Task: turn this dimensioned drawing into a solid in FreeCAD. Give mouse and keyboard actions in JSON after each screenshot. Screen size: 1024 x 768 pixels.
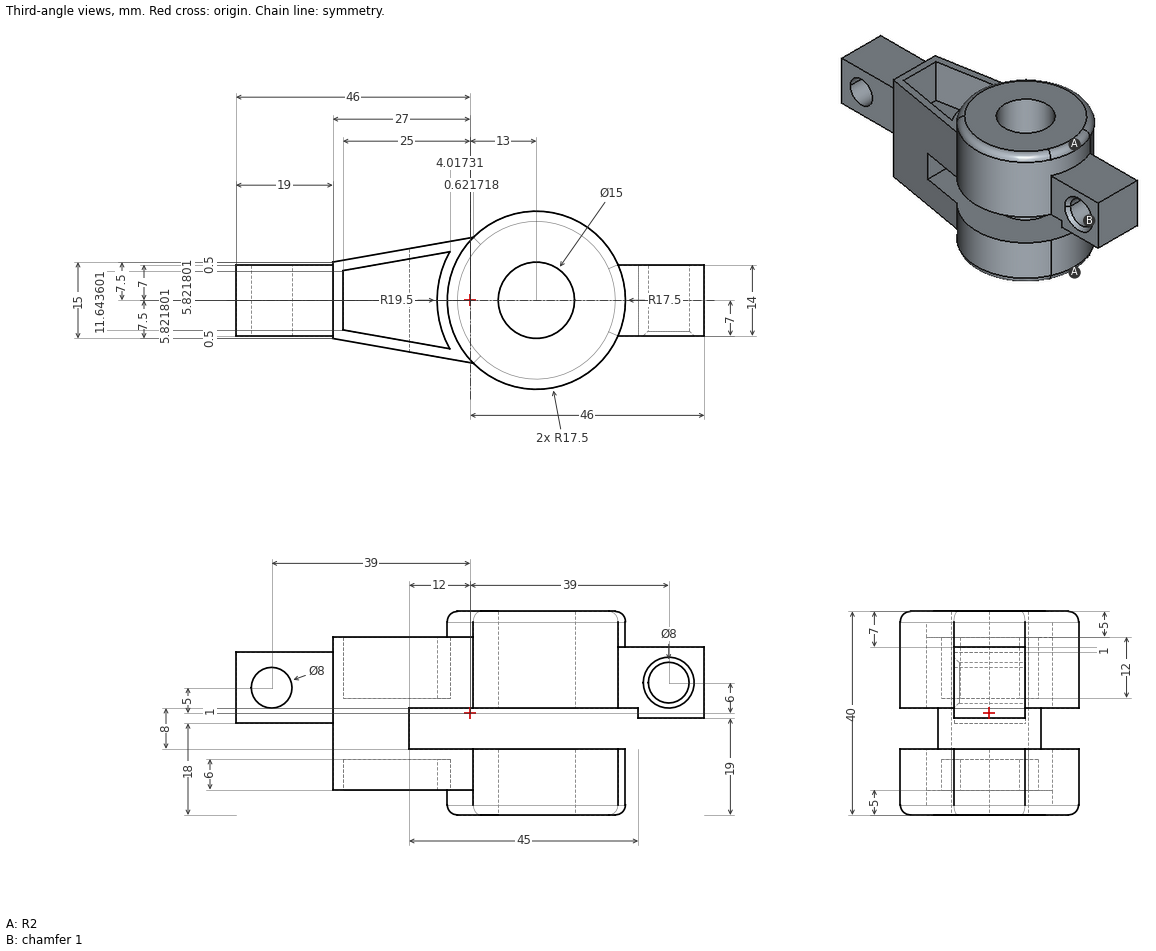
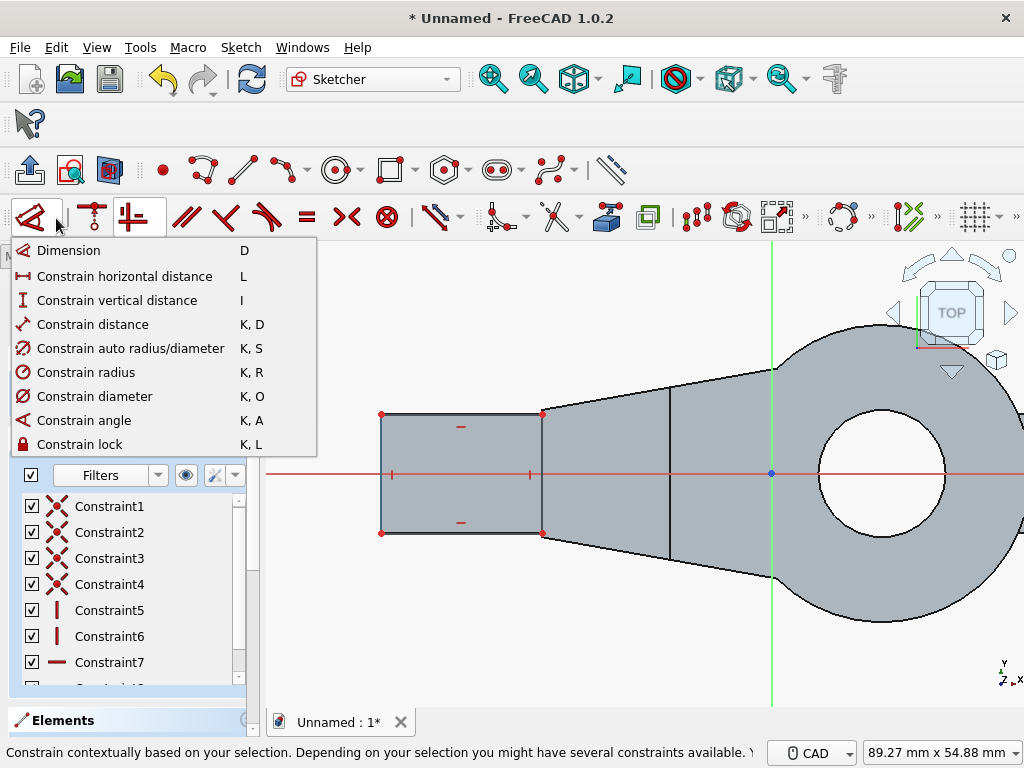
{"action": "left_click", "coordinate": [164, 300]}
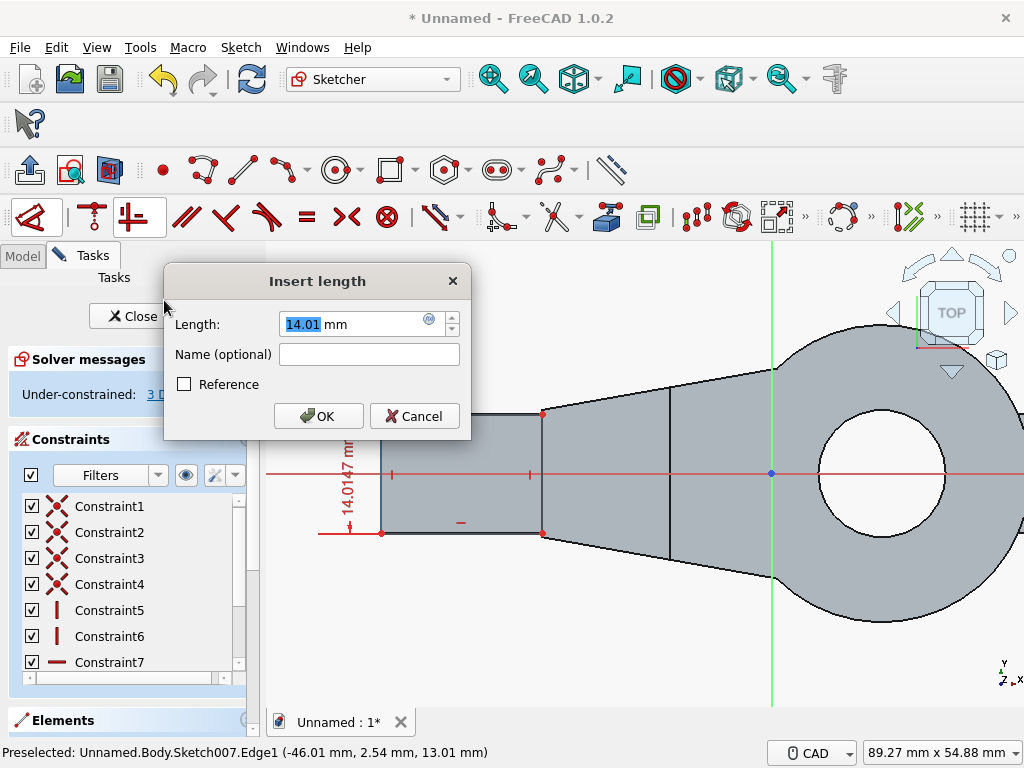
{"action": "type", "text": "14"}
{"action": "key", "text": "Return"}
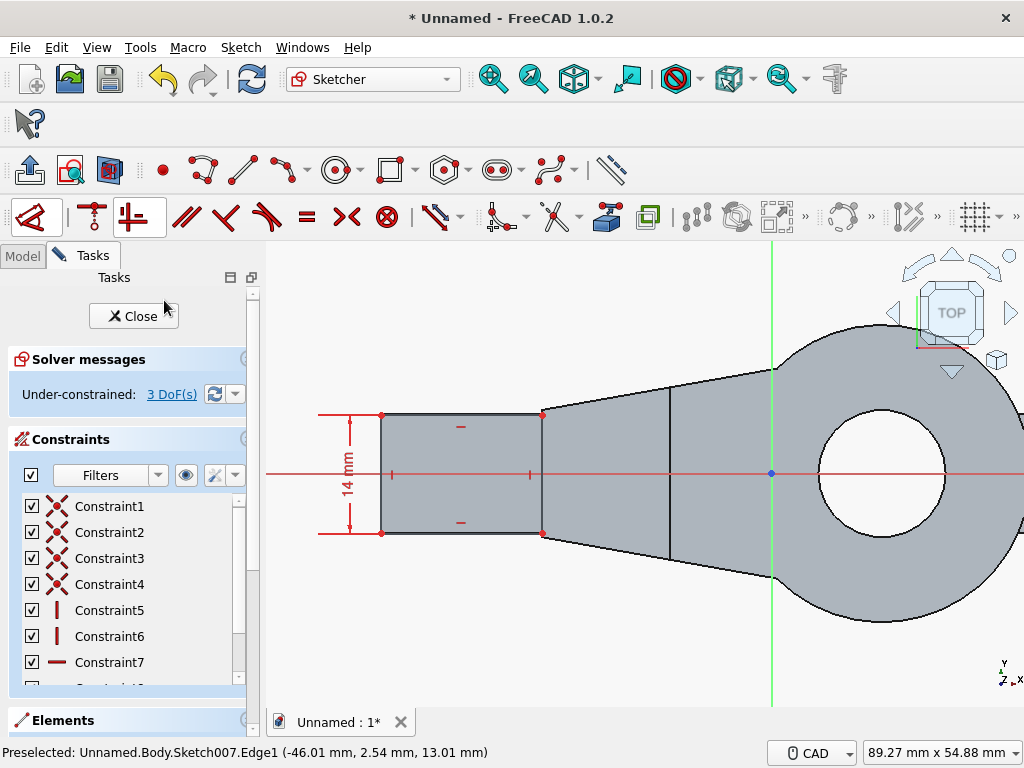
{"action": "left_click", "coordinate": [429, 534]}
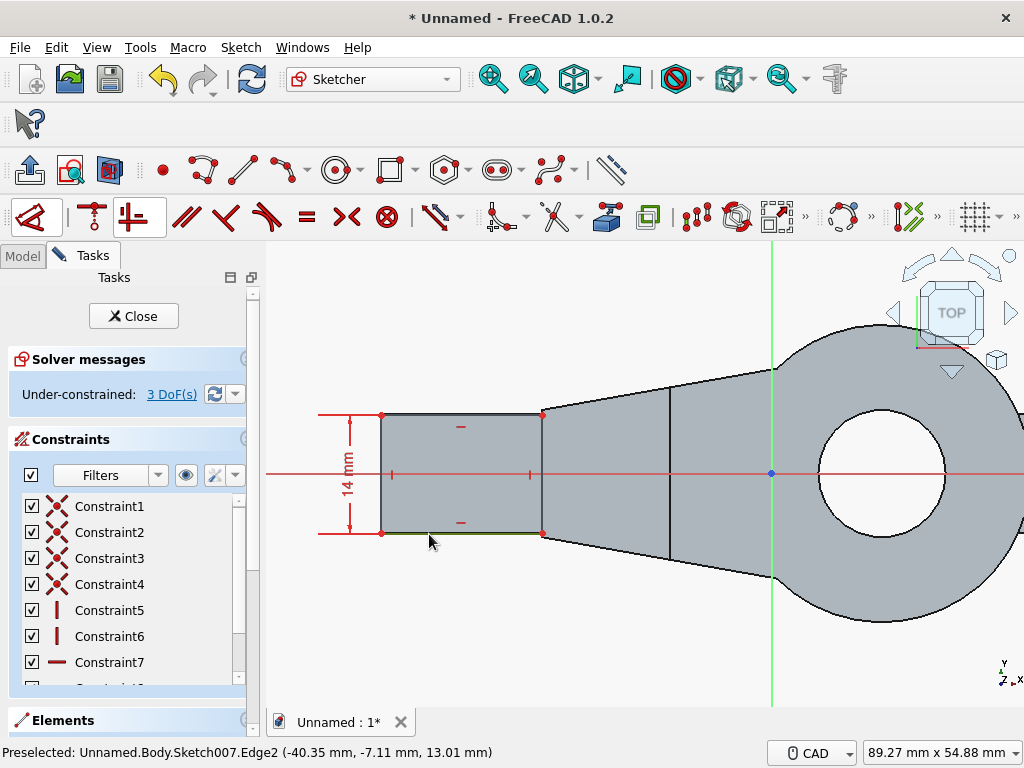
{"action": "key", "text": "l"}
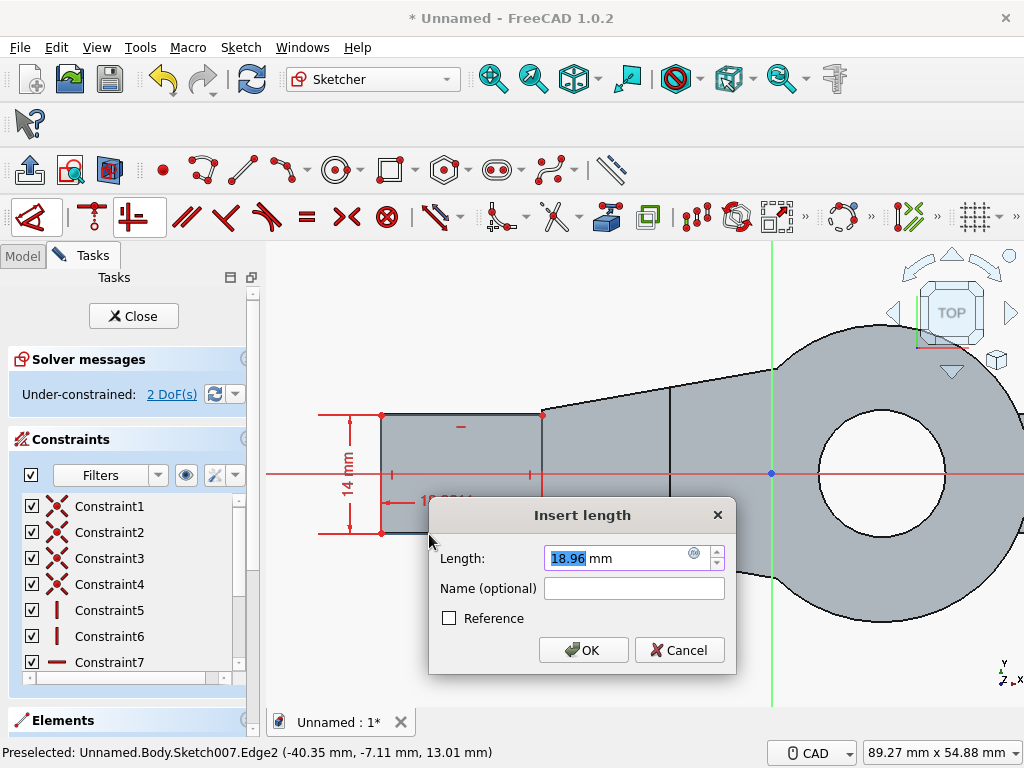
{"action": "type", "text": "19"}
{"action": "key", "text": "Return"}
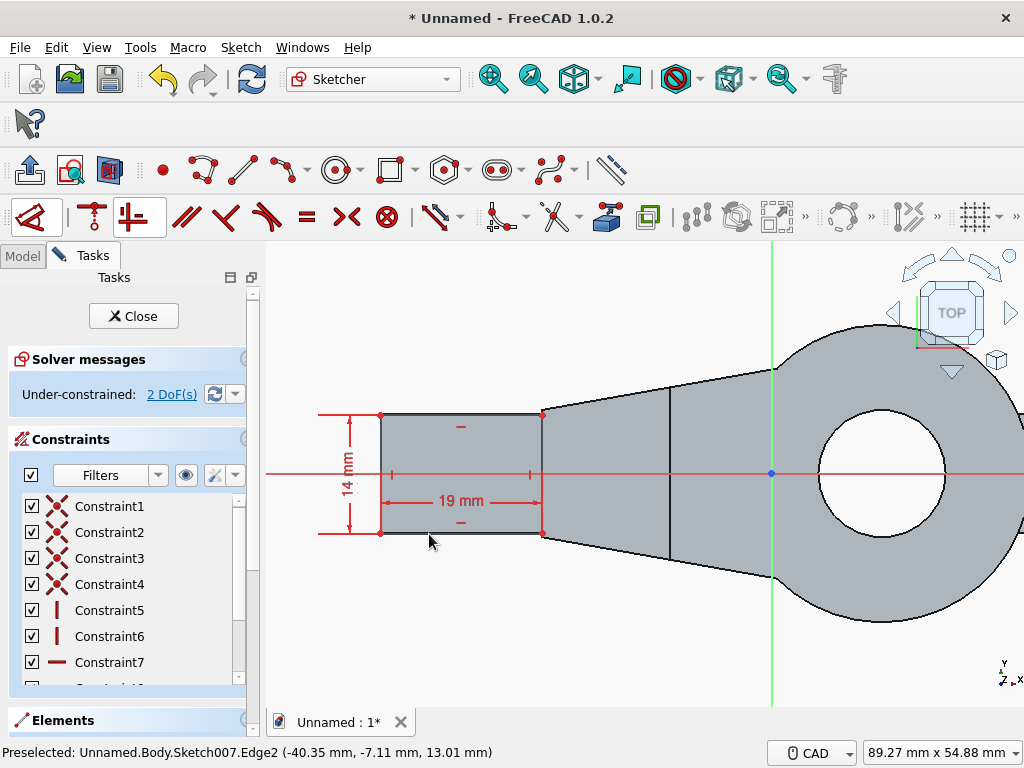
{"action": "left_click", "coordinate": [381, 415]}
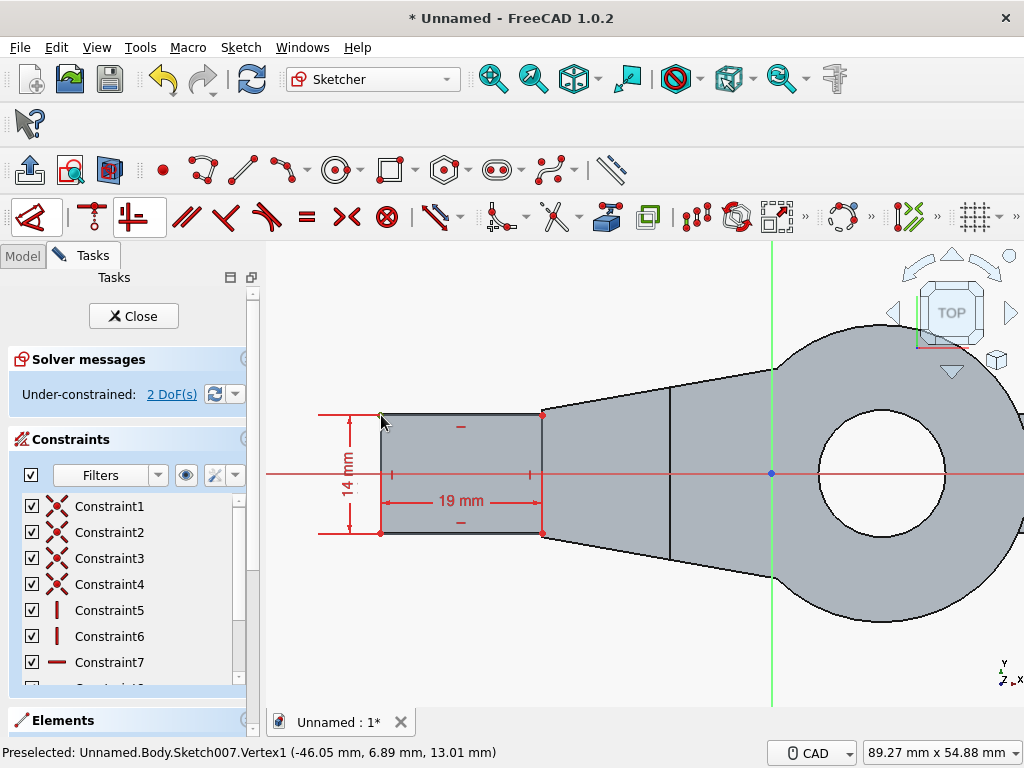
{"action": "left_click", "coordinate": [56, 218]}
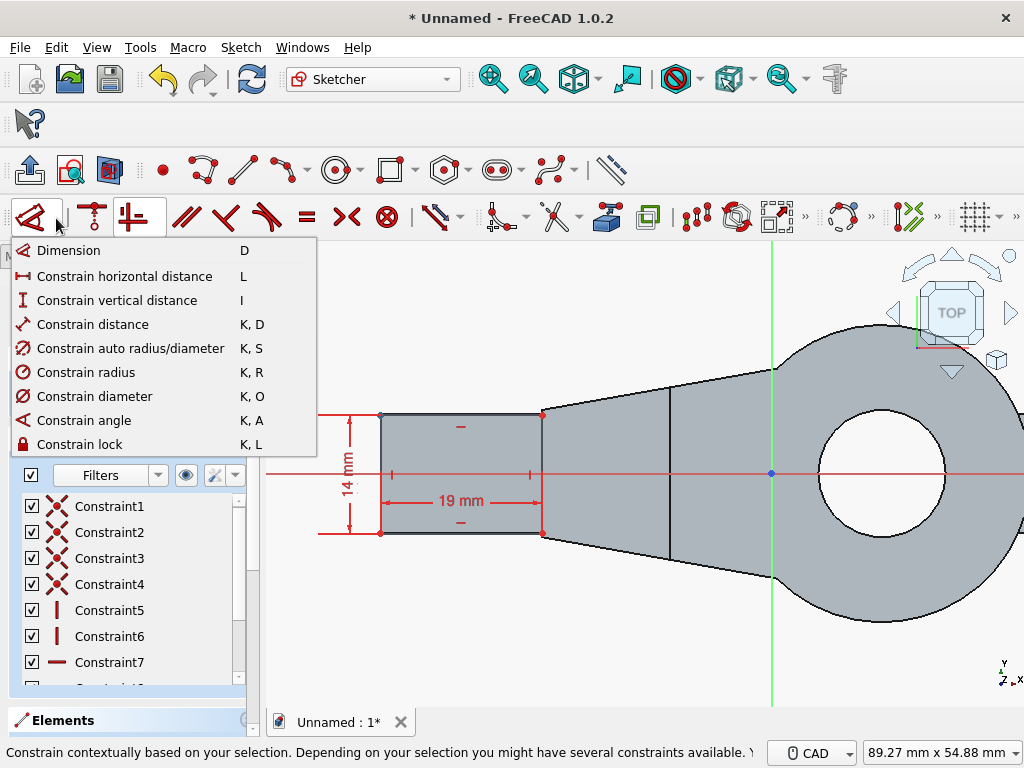
{"action": "left_click", "coordinate": [164, 300]}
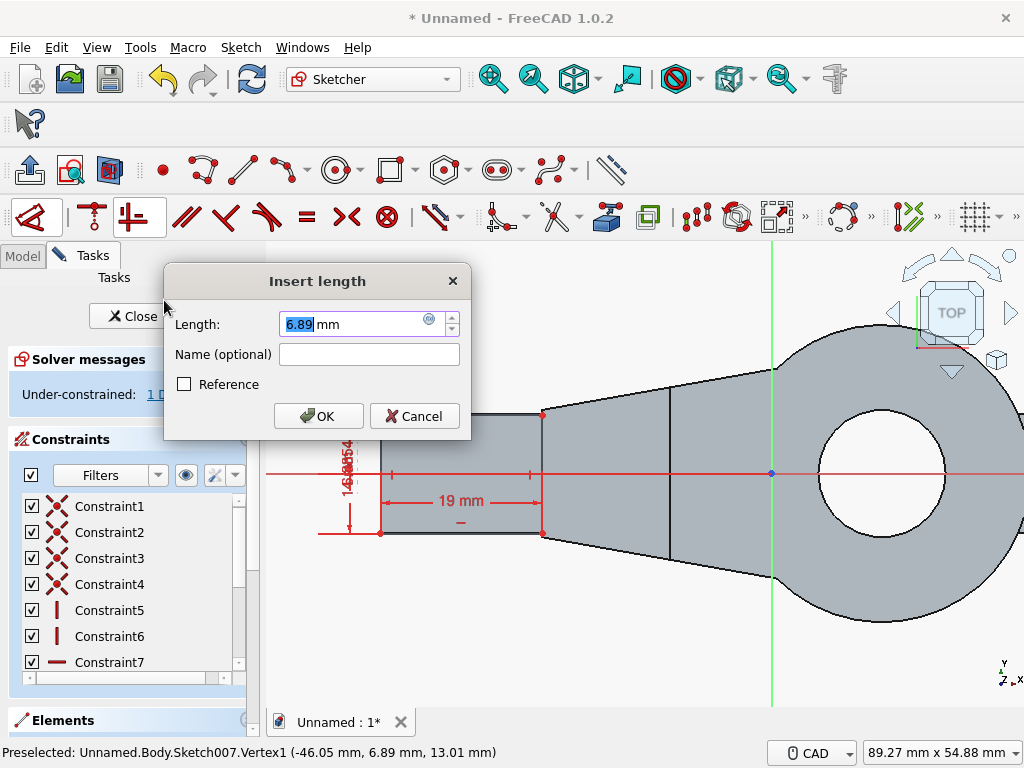
{"action": "type", "text": "7"}
{"action": "key", "text": "Return"}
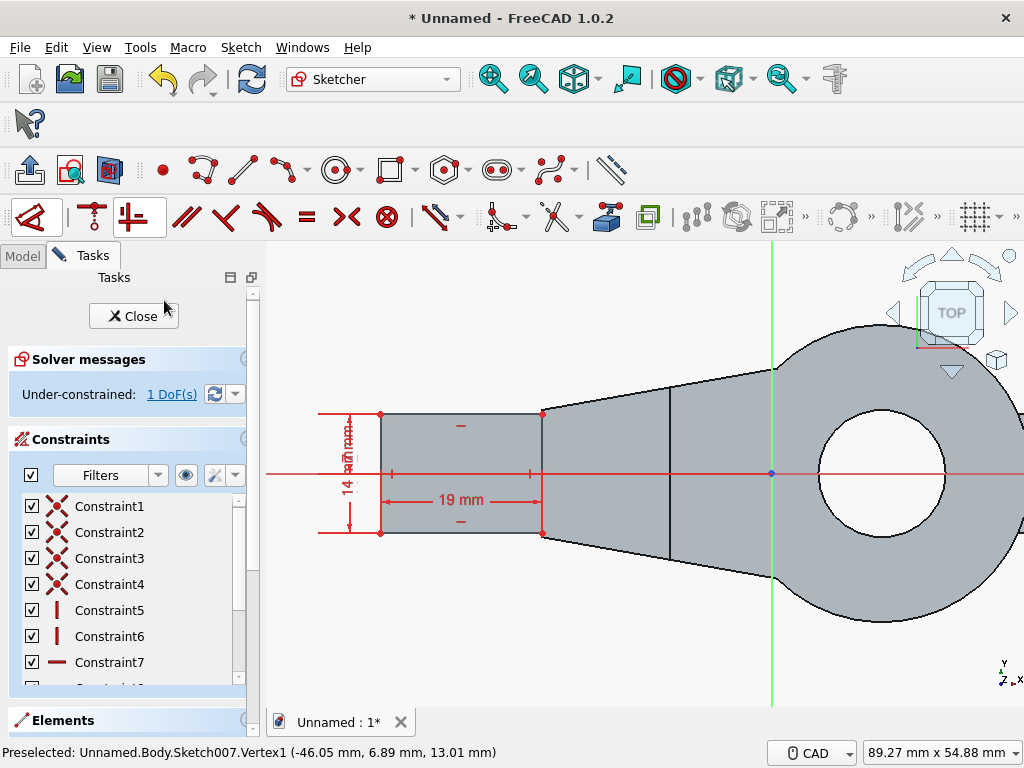
{"action": "left_click", "coordinate": [381, 414]}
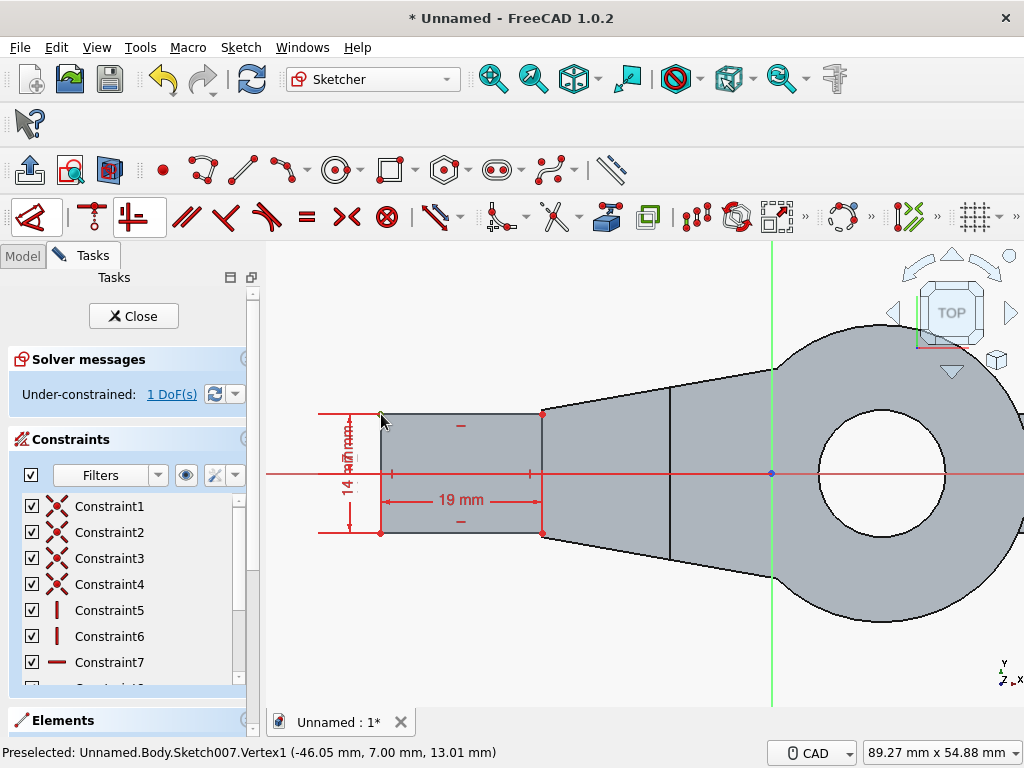
{"action": "key", "text": "l"}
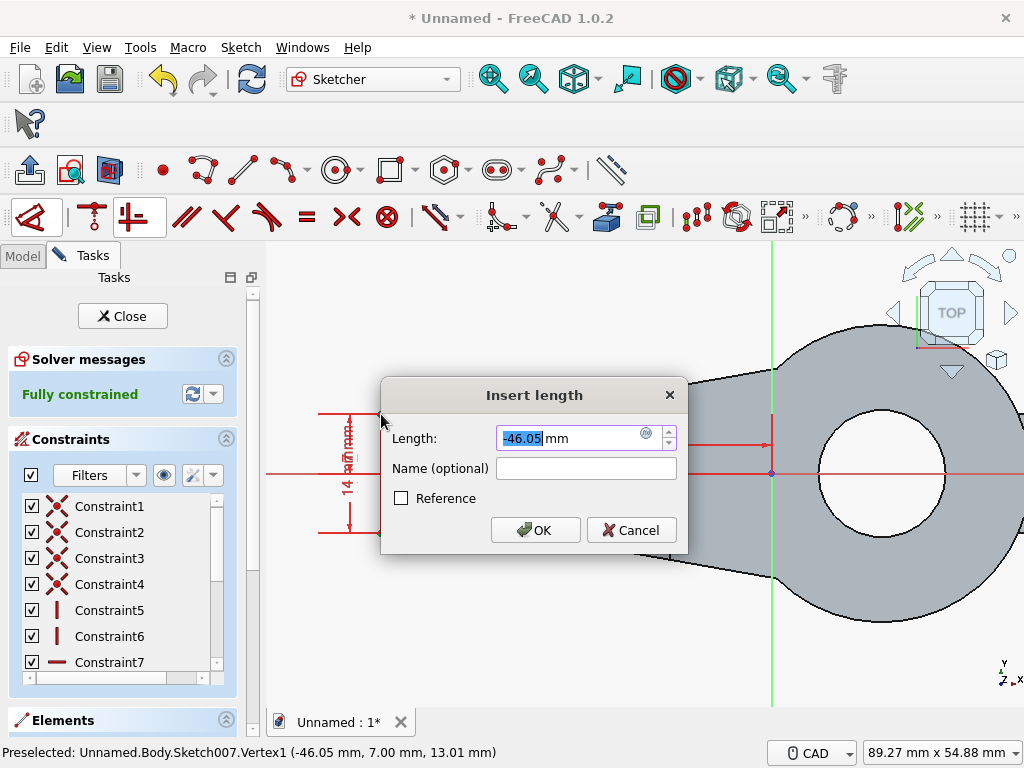
{"action": "type", "text": "-46"}
{"action": "key", "text": "Return"}